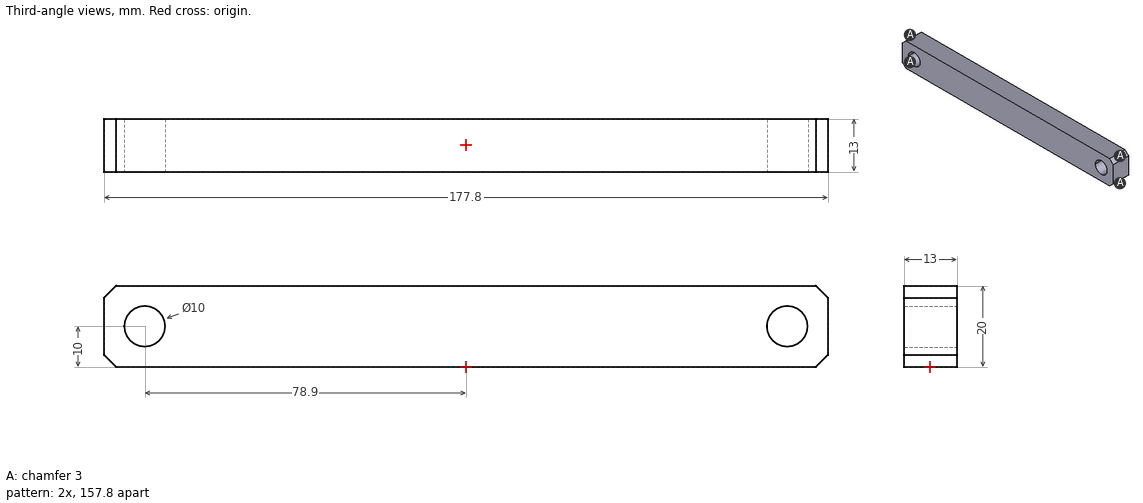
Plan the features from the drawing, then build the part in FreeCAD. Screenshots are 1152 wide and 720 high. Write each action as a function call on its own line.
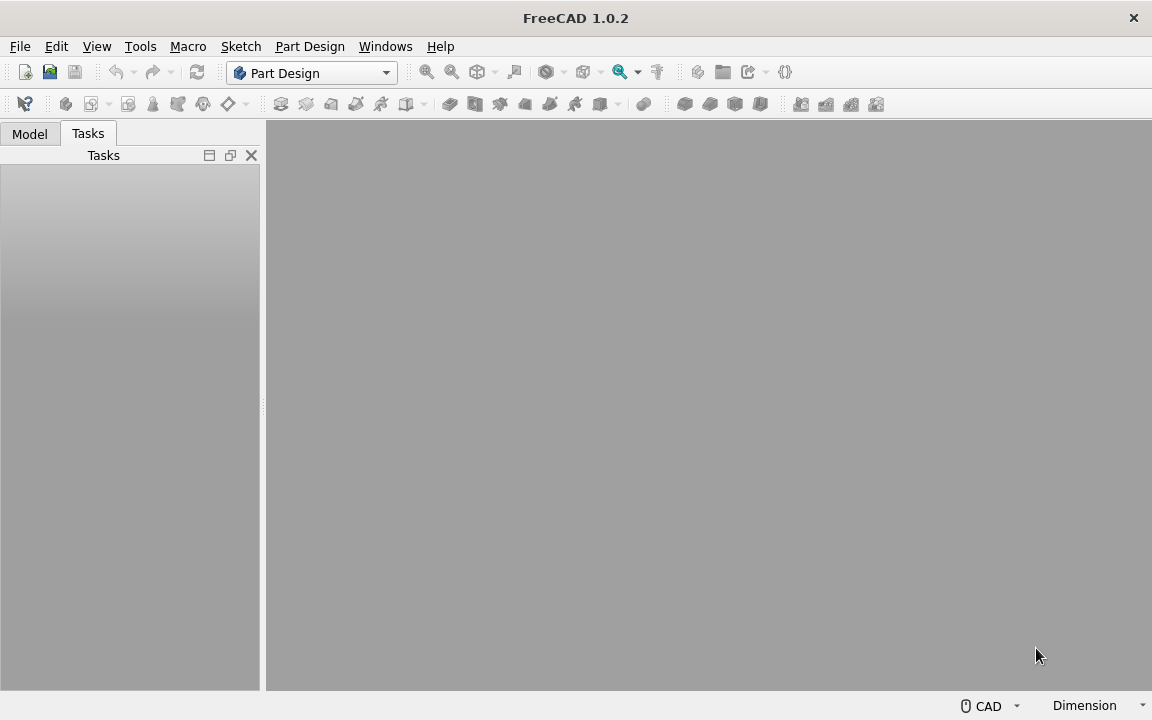
click(25, 72)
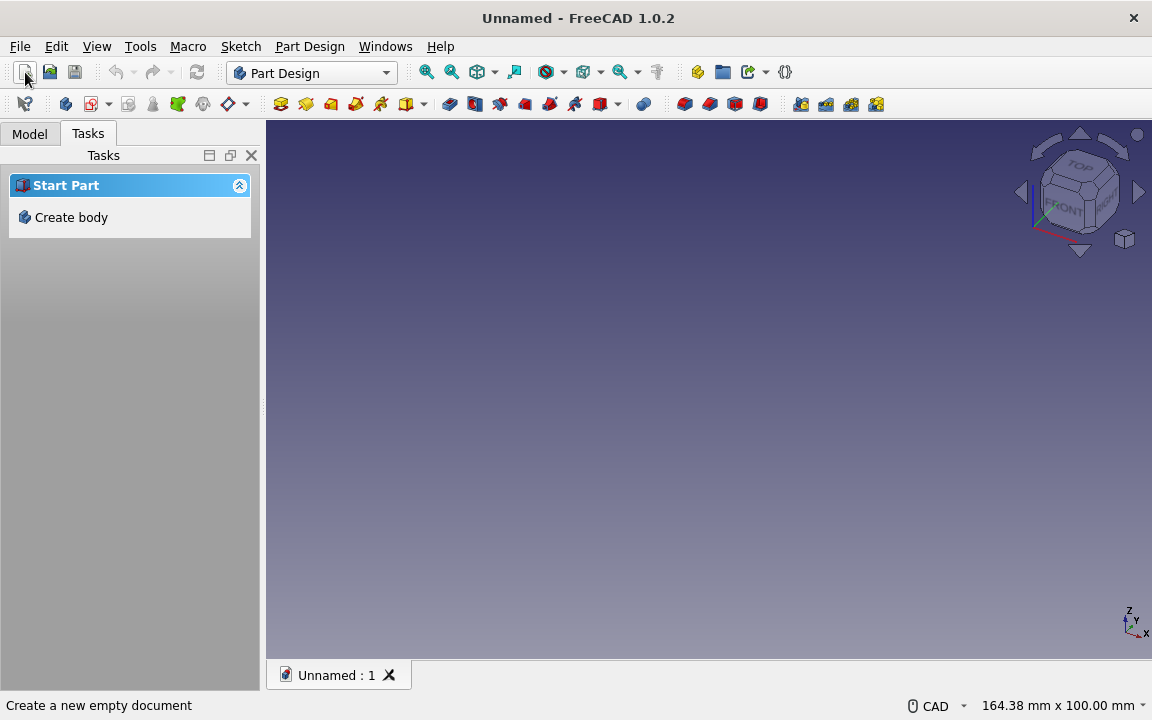
click(90, 104)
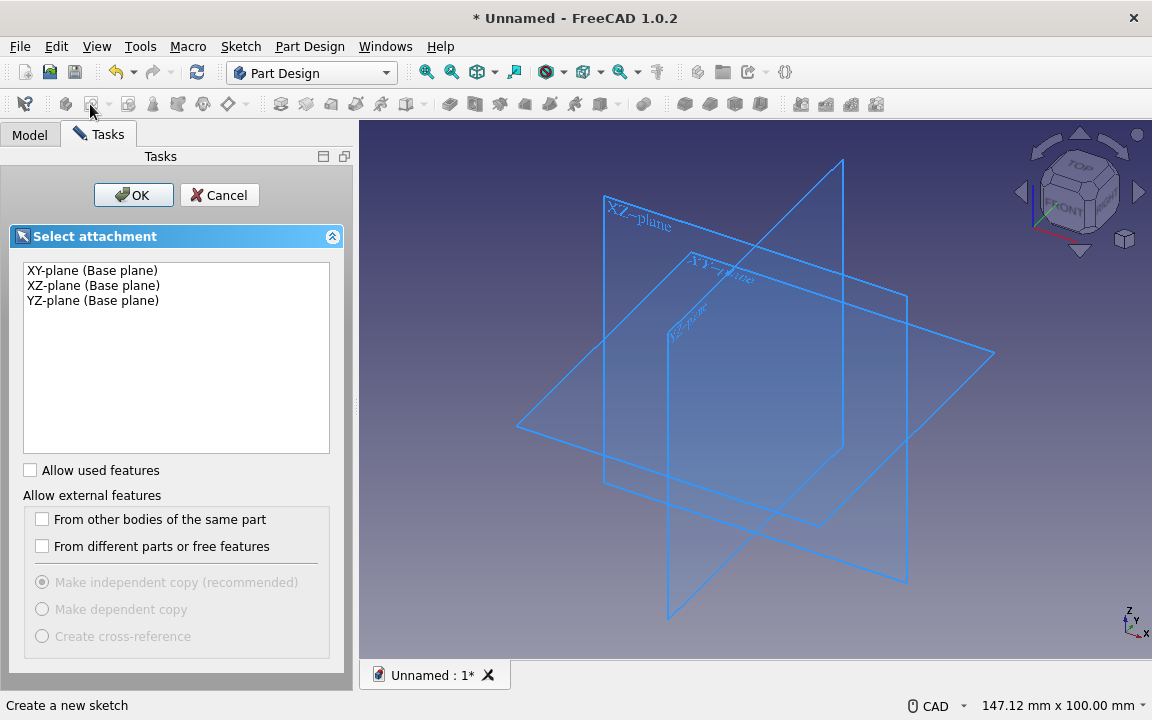
click(84, 270)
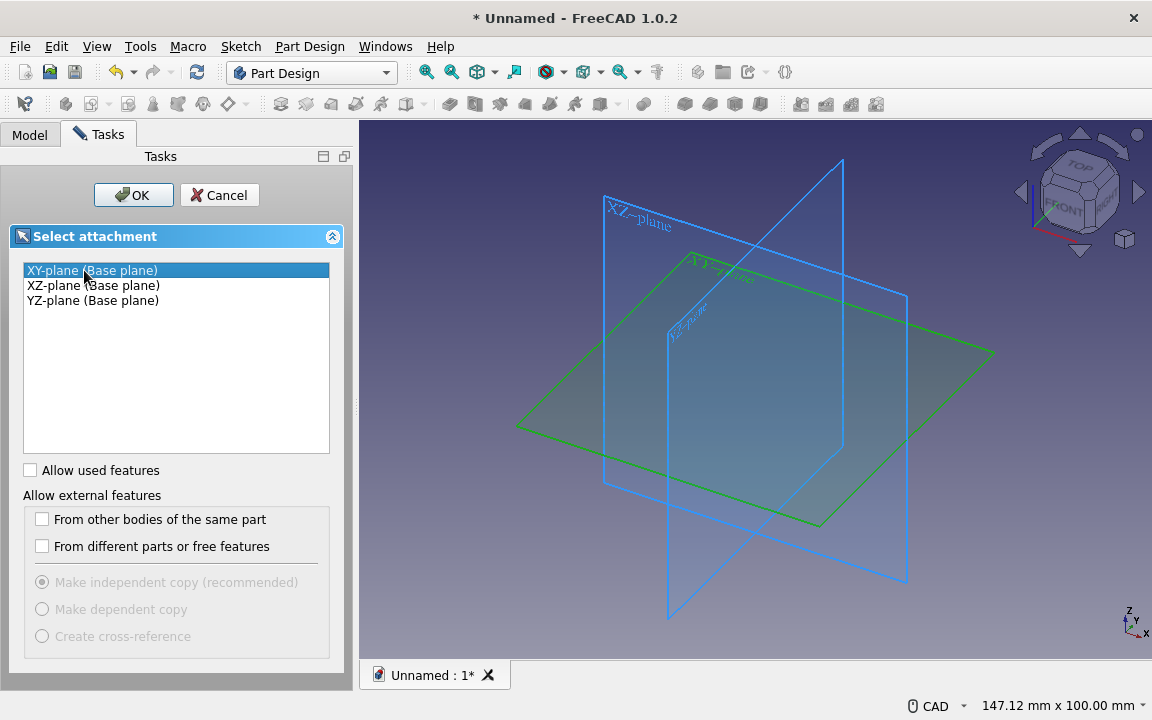
click(134, 195)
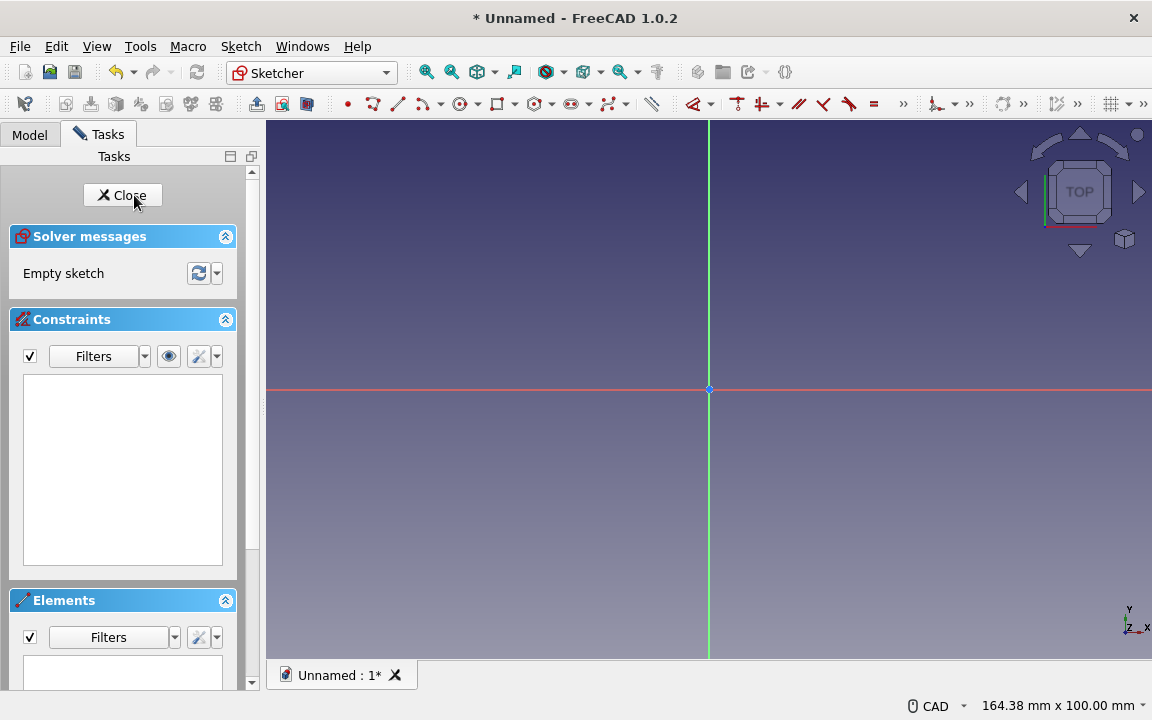
scroll(557, 390, down, 3)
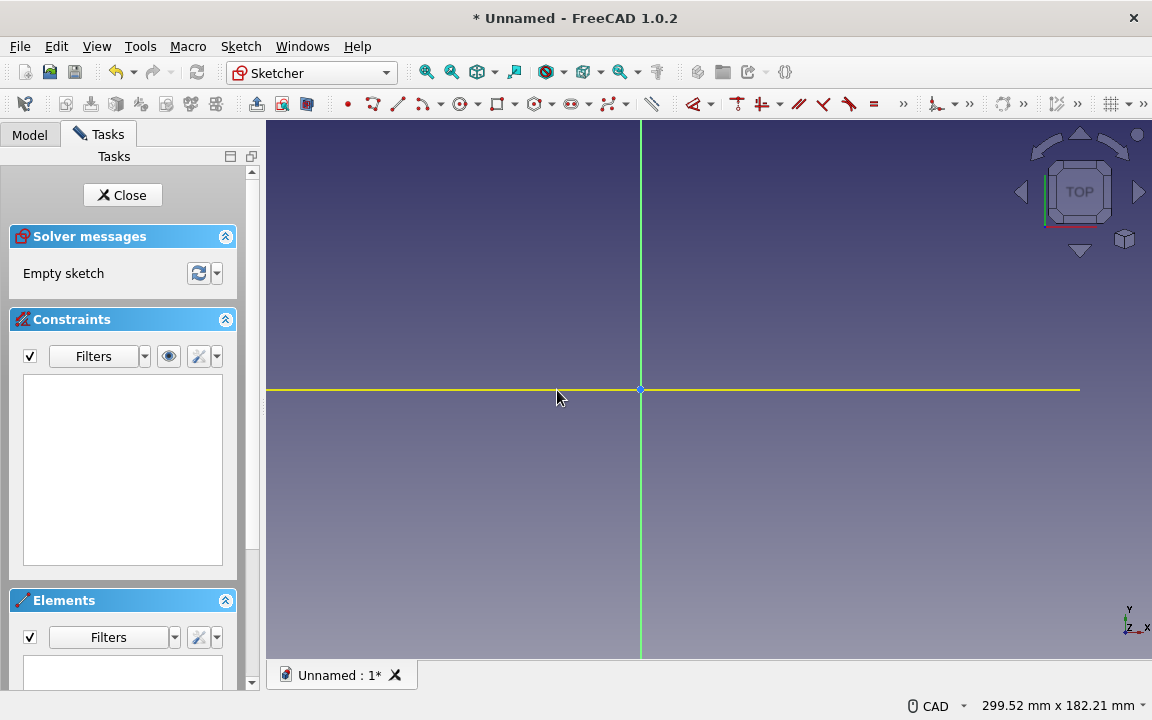
click(514, 104)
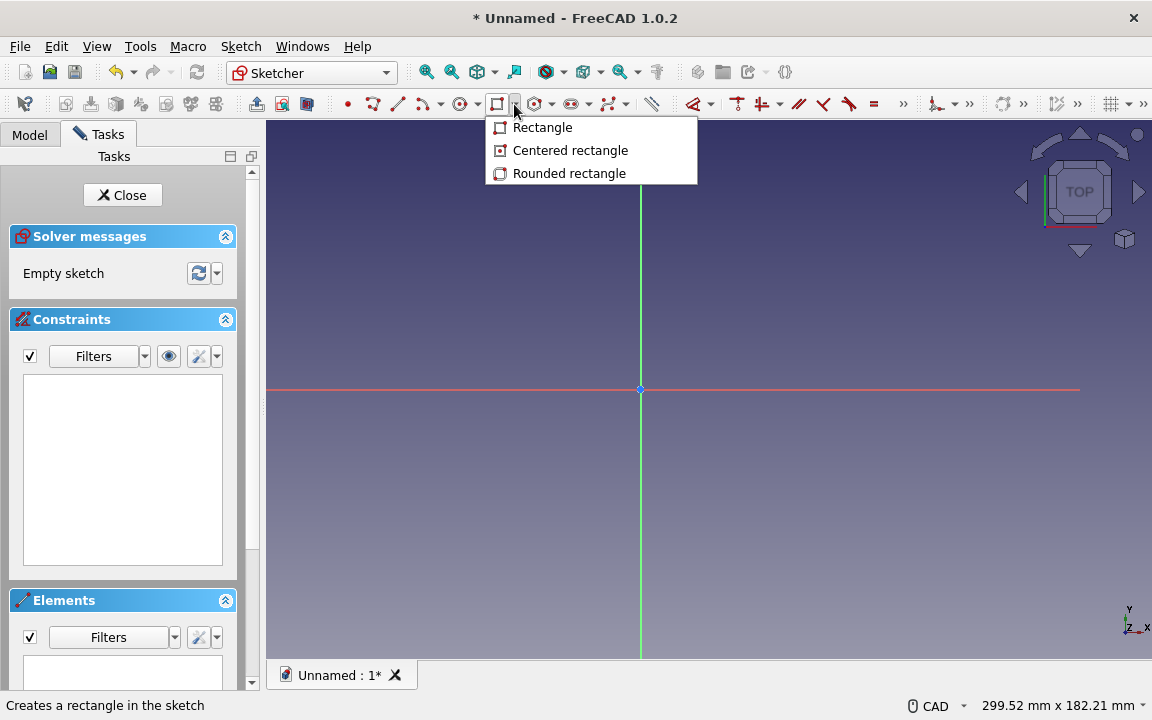
click(592, 150)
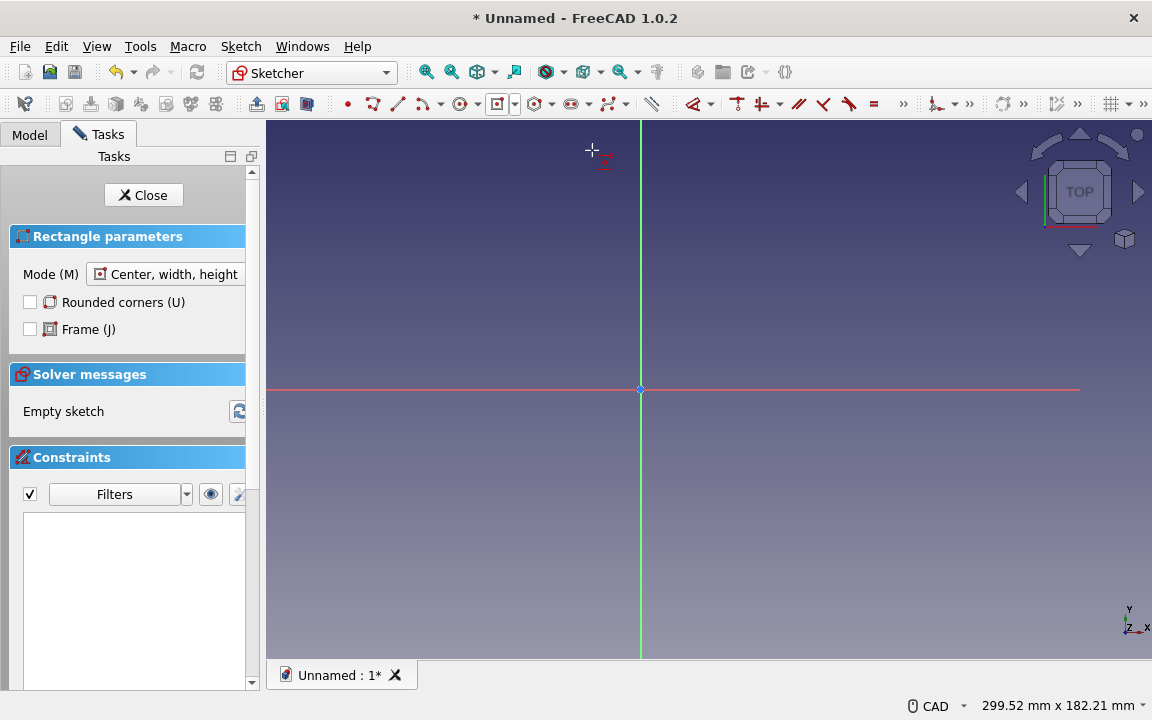
click(641, 390)
click(904, 371)
key(Escape)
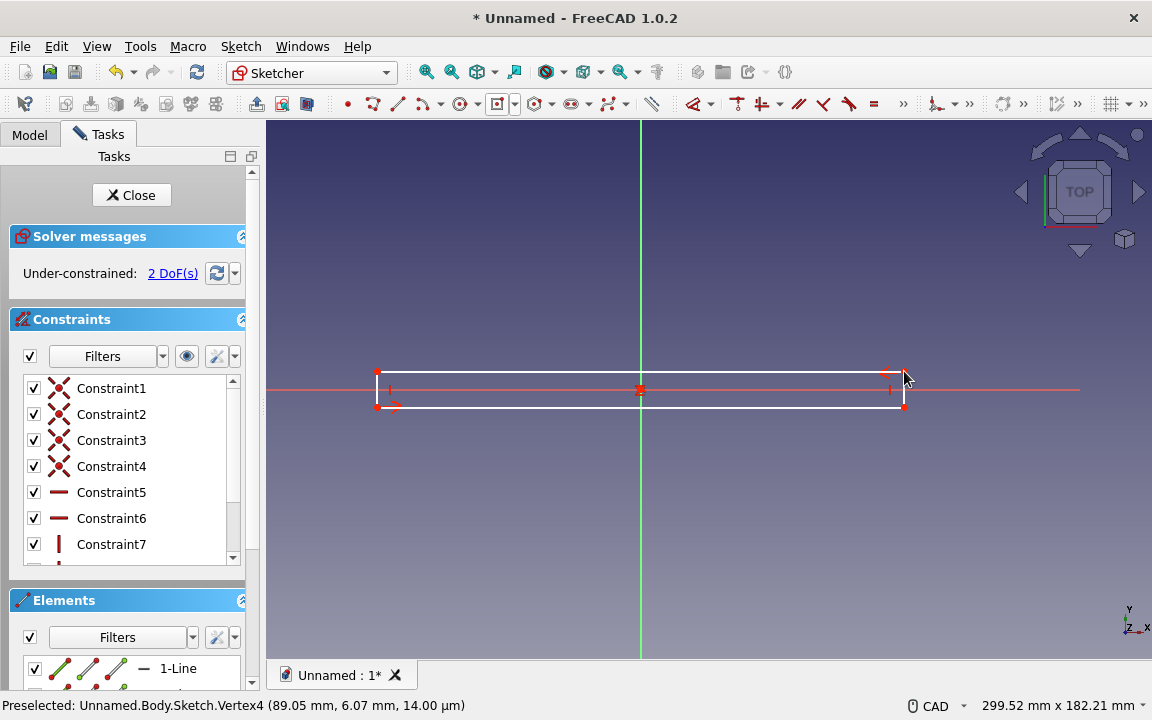
click(904, 394)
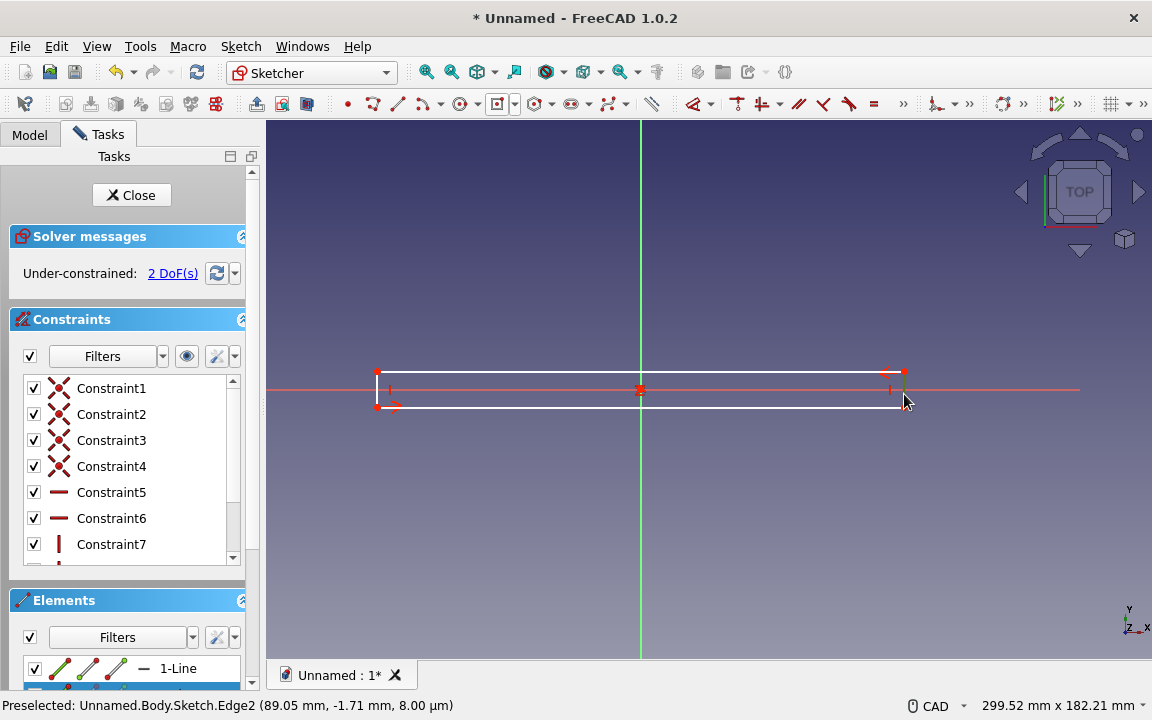
click(710, 104)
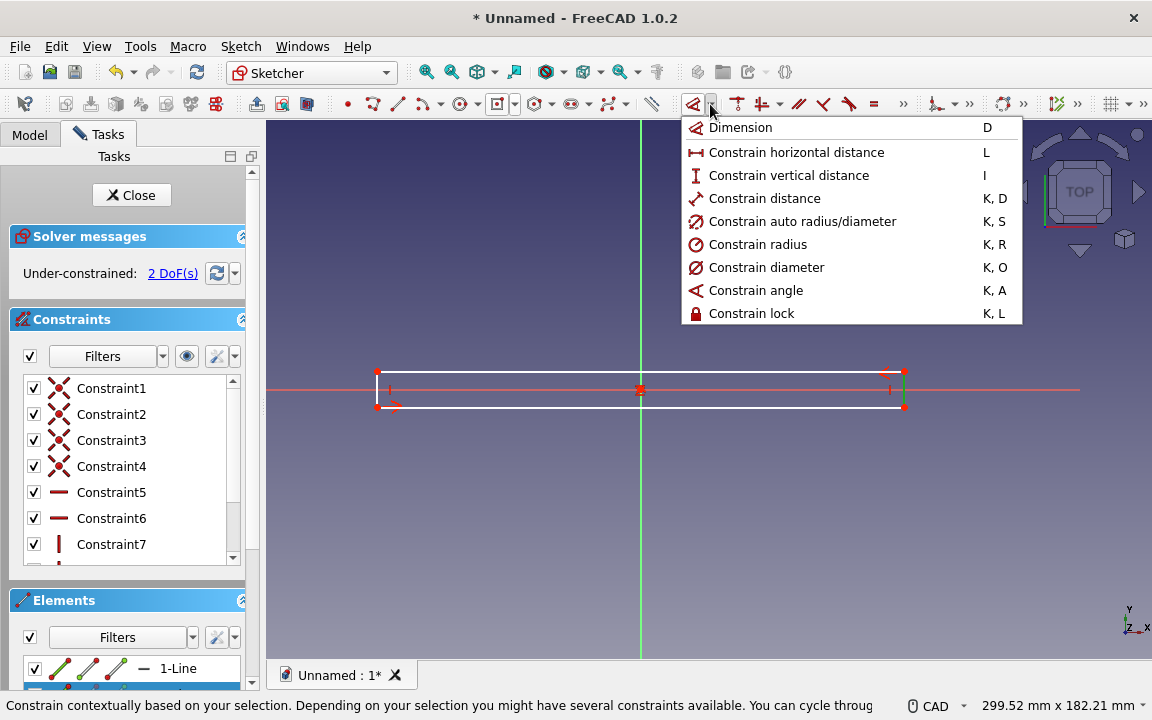
click(852, 176)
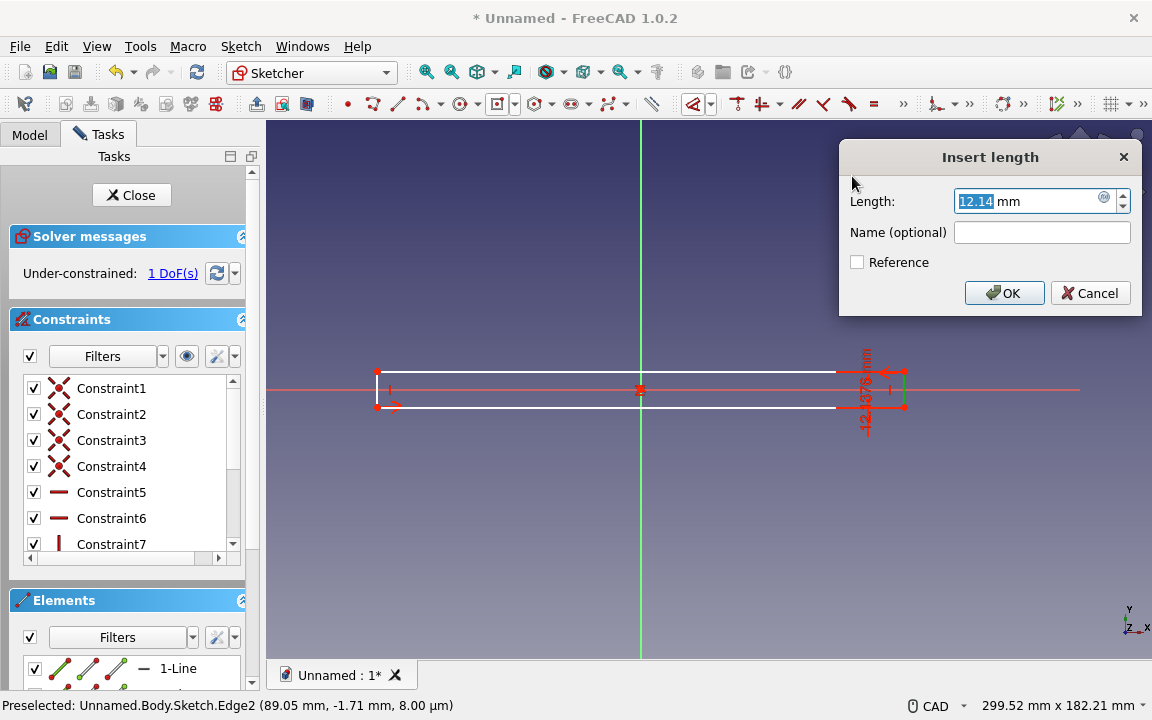
text(13)
key(Return)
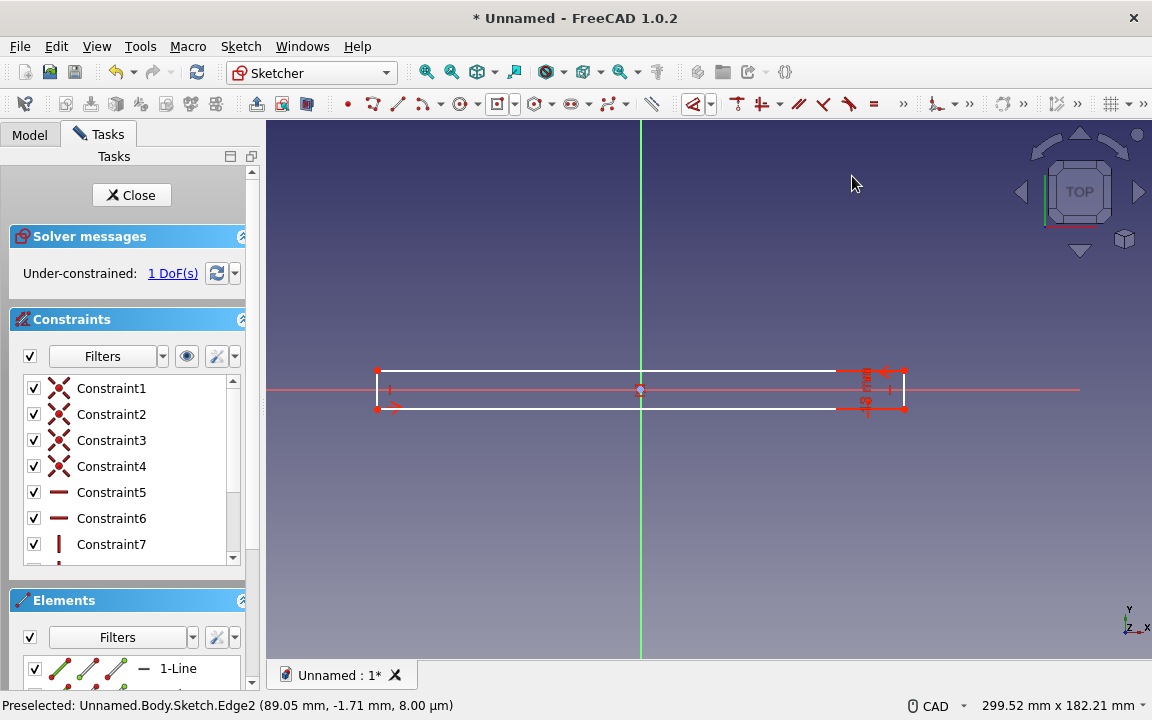
click(535, 409)